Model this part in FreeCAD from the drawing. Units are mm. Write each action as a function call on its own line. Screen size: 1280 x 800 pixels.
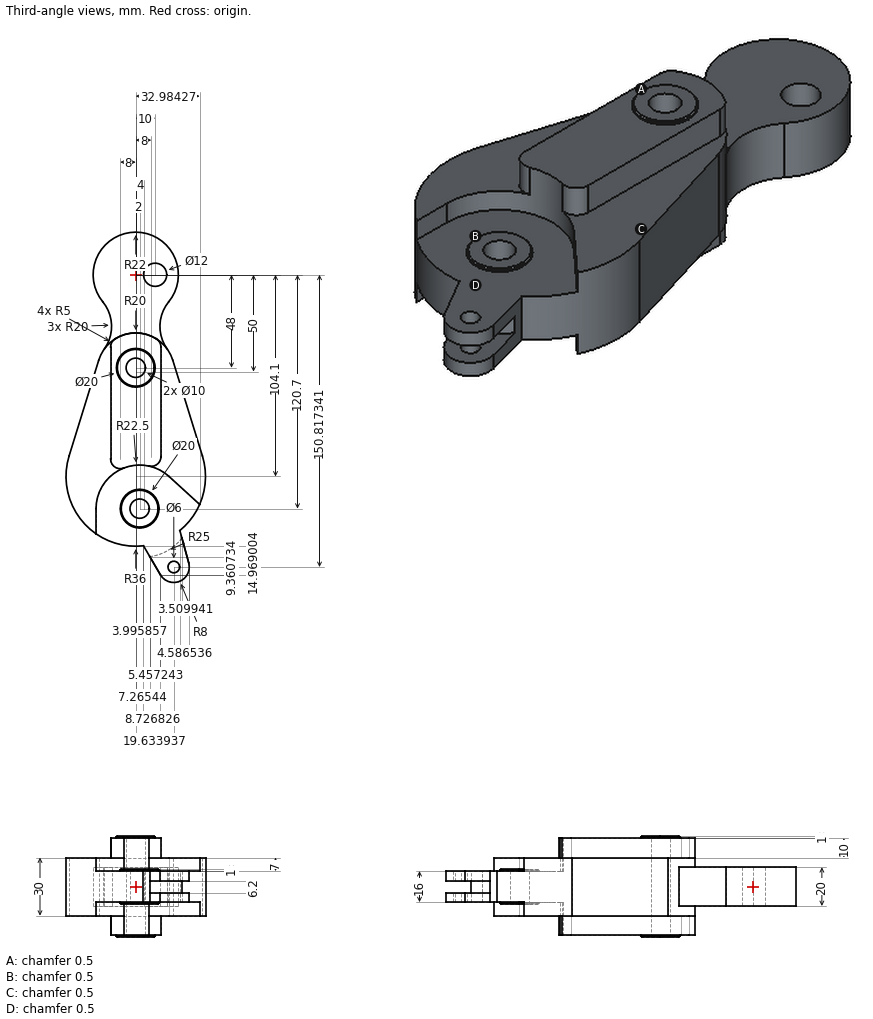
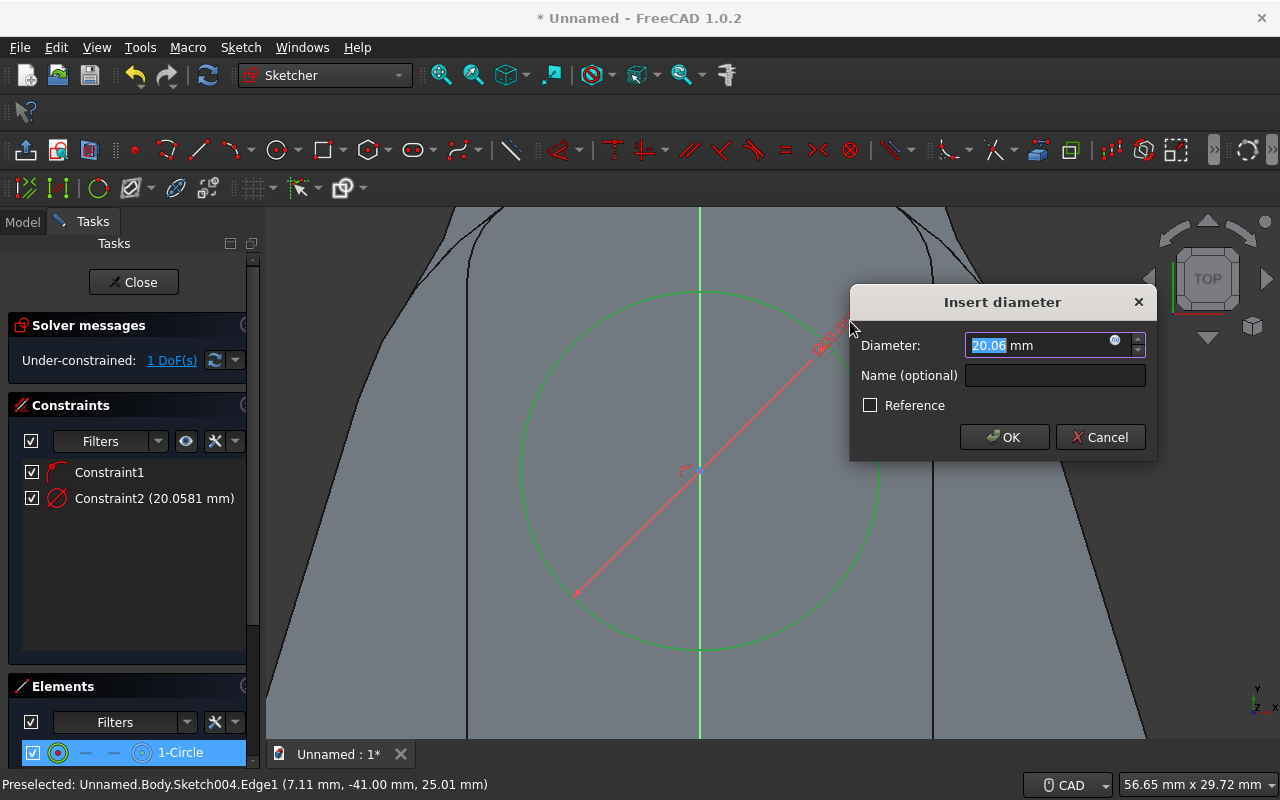
text(20)
key(Return)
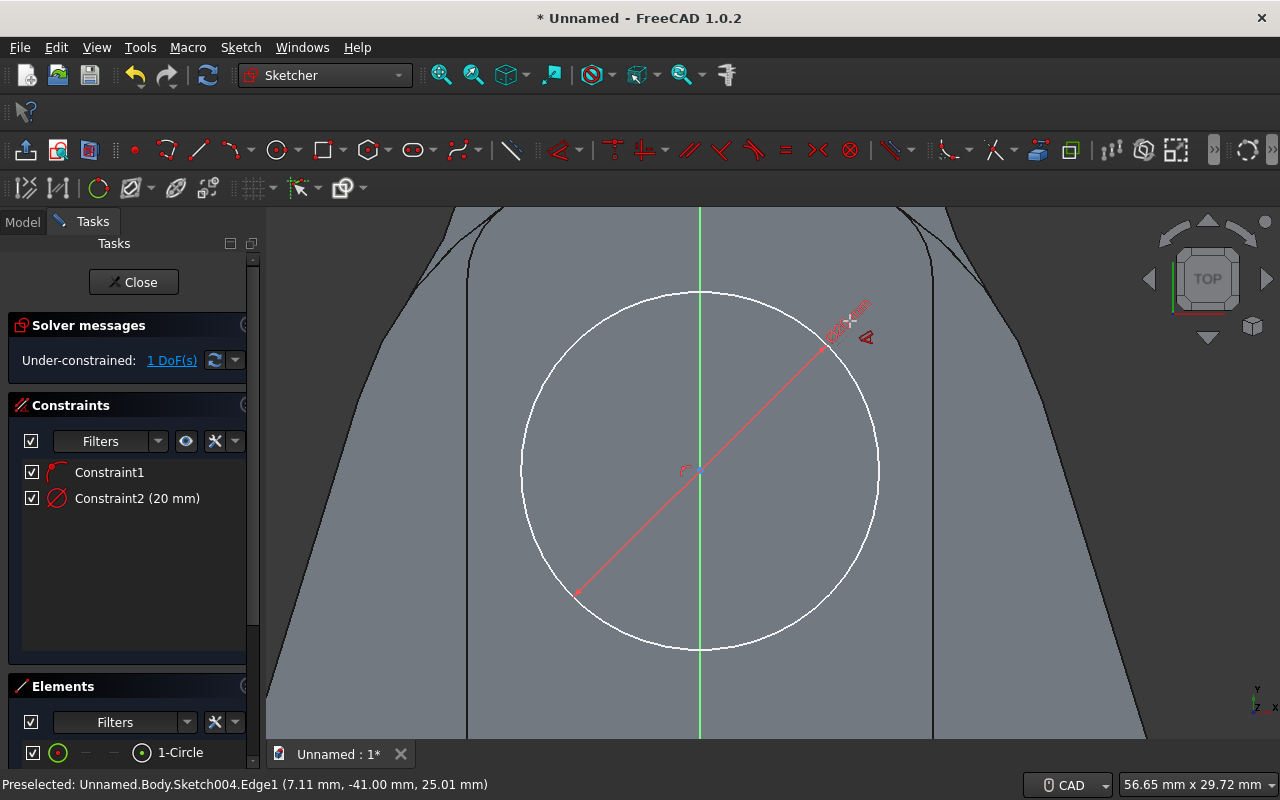
click(700, 471)
click(734, 353)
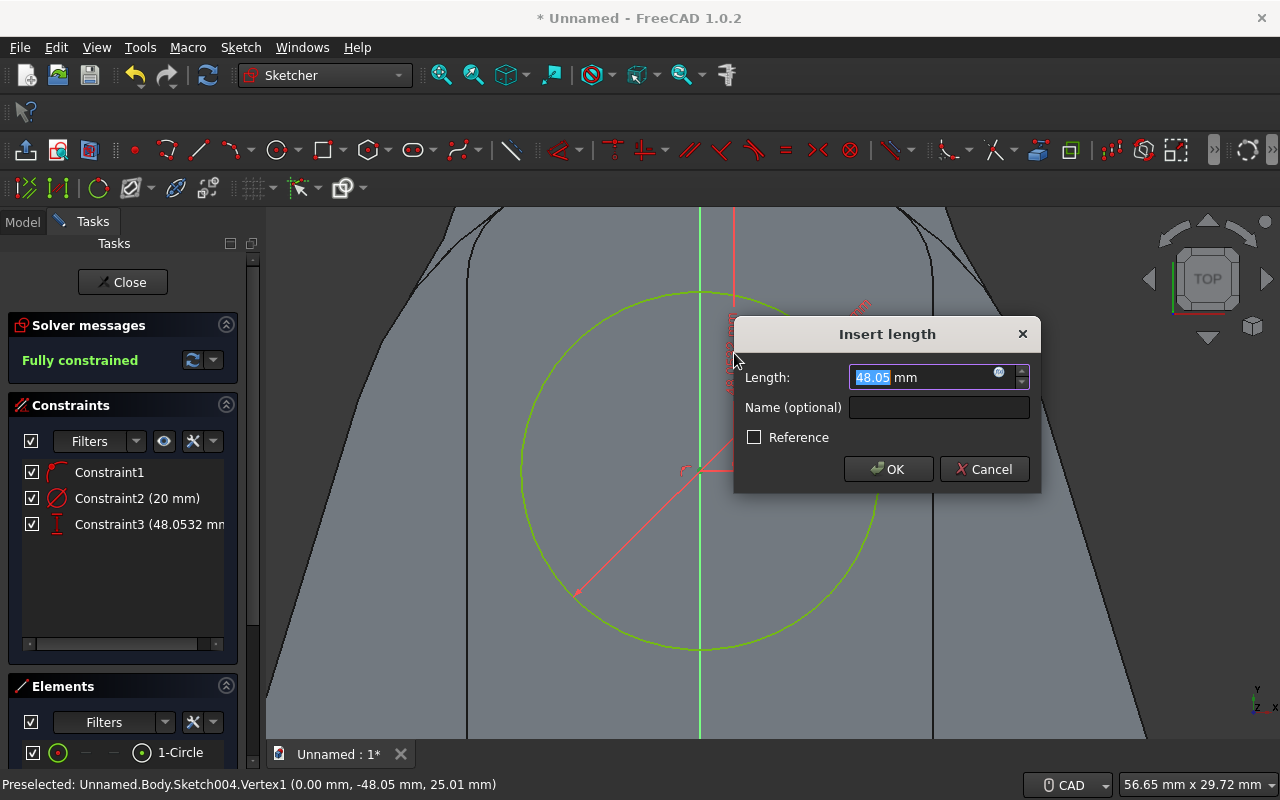
text(48)
key(Return)
key(Escape)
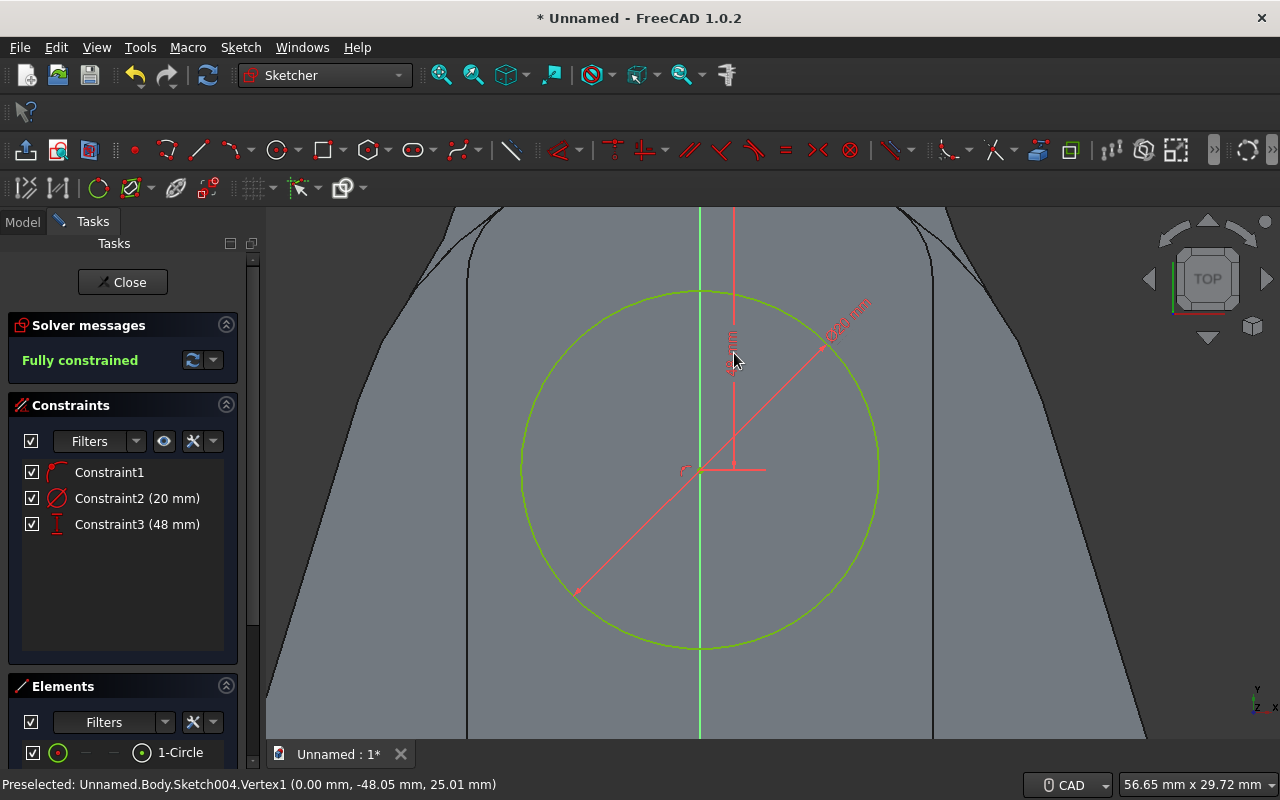
click(123, 282)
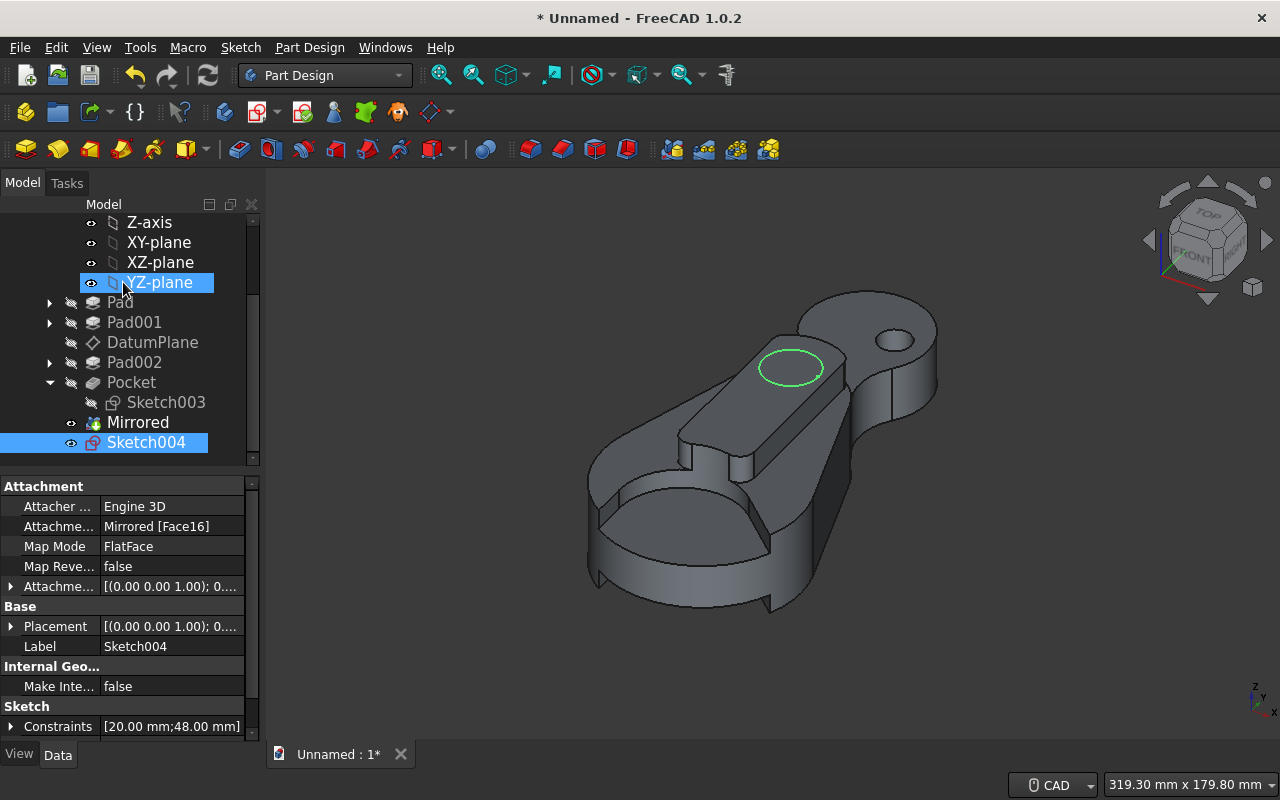
click(26, 150)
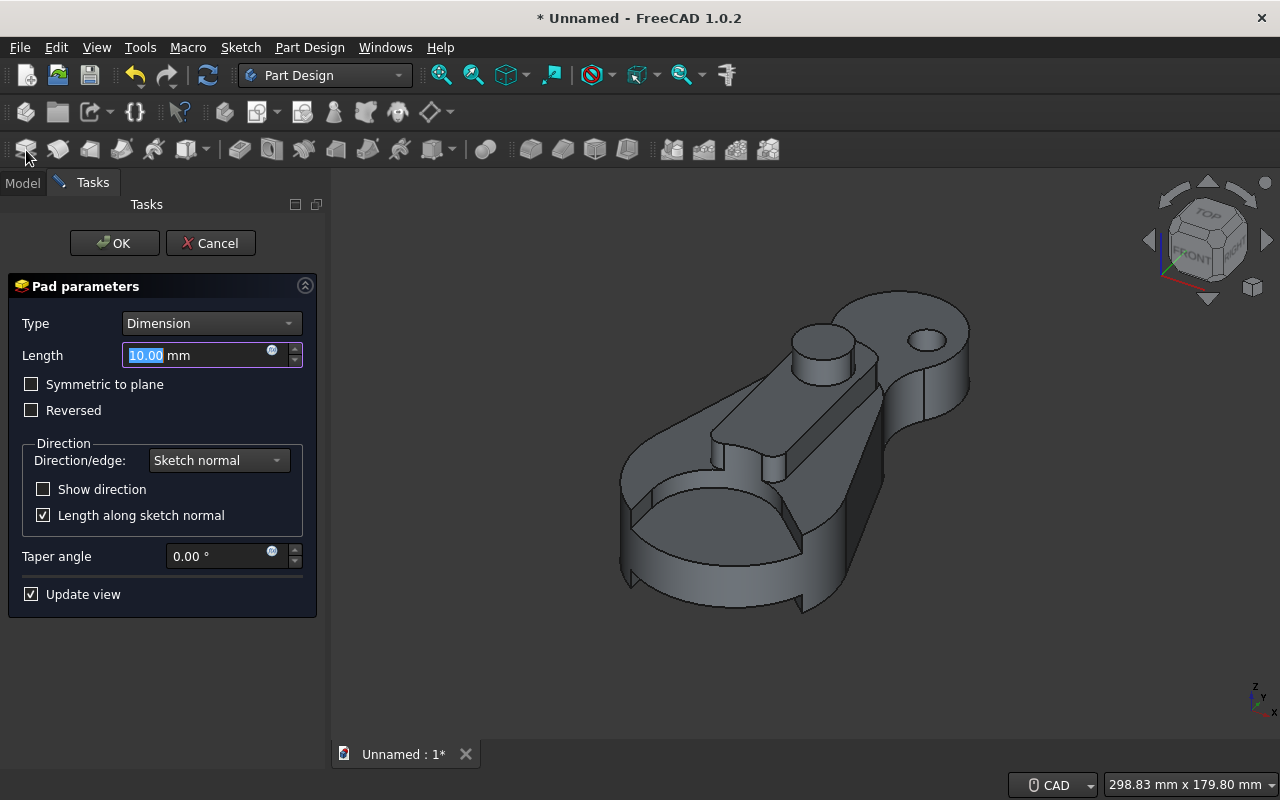
text(1)
key(Tab)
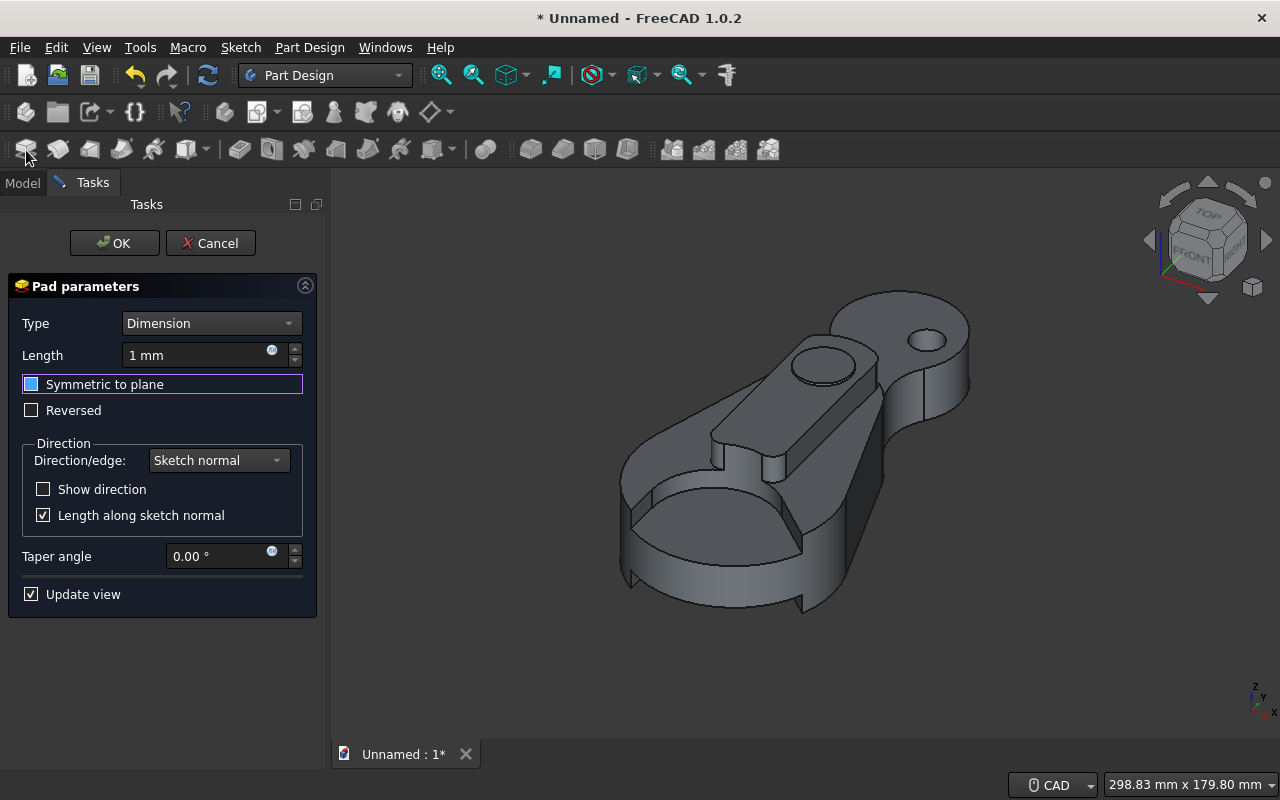
click(115, 243)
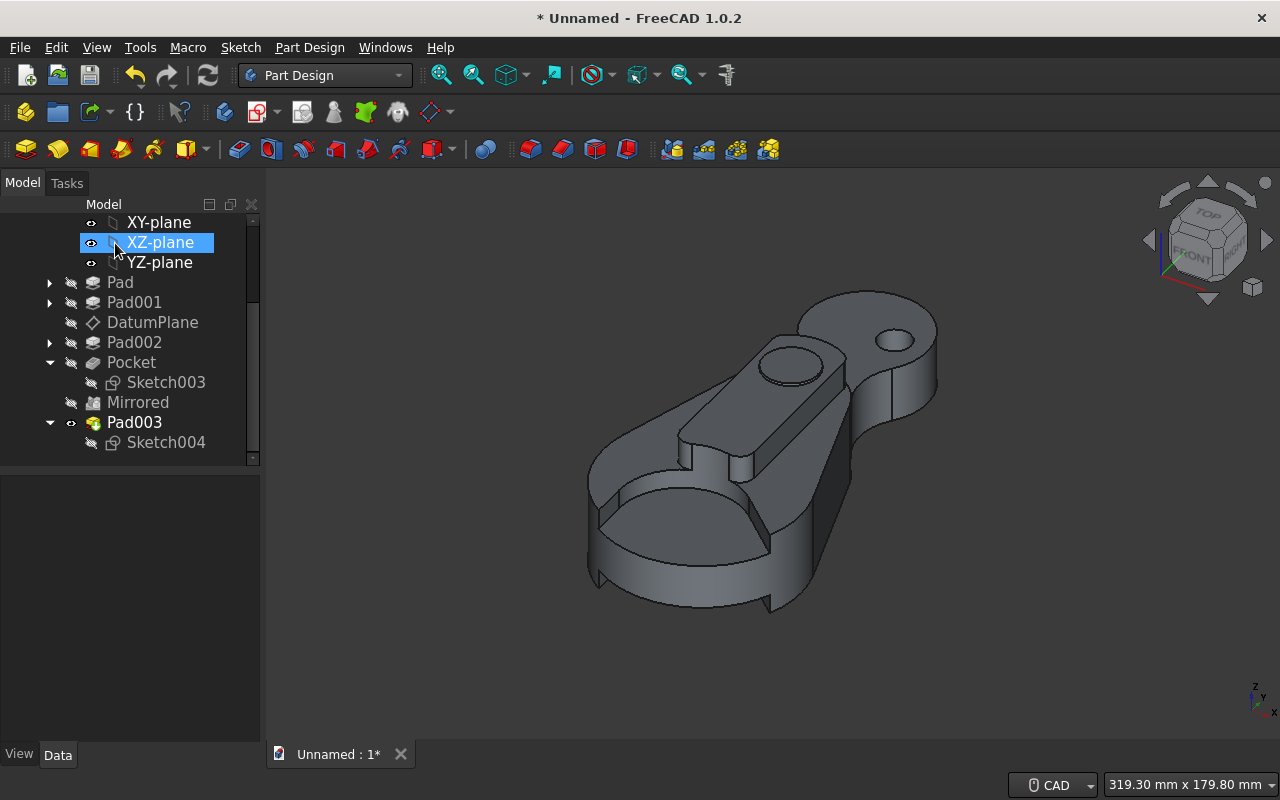
click(759, 366)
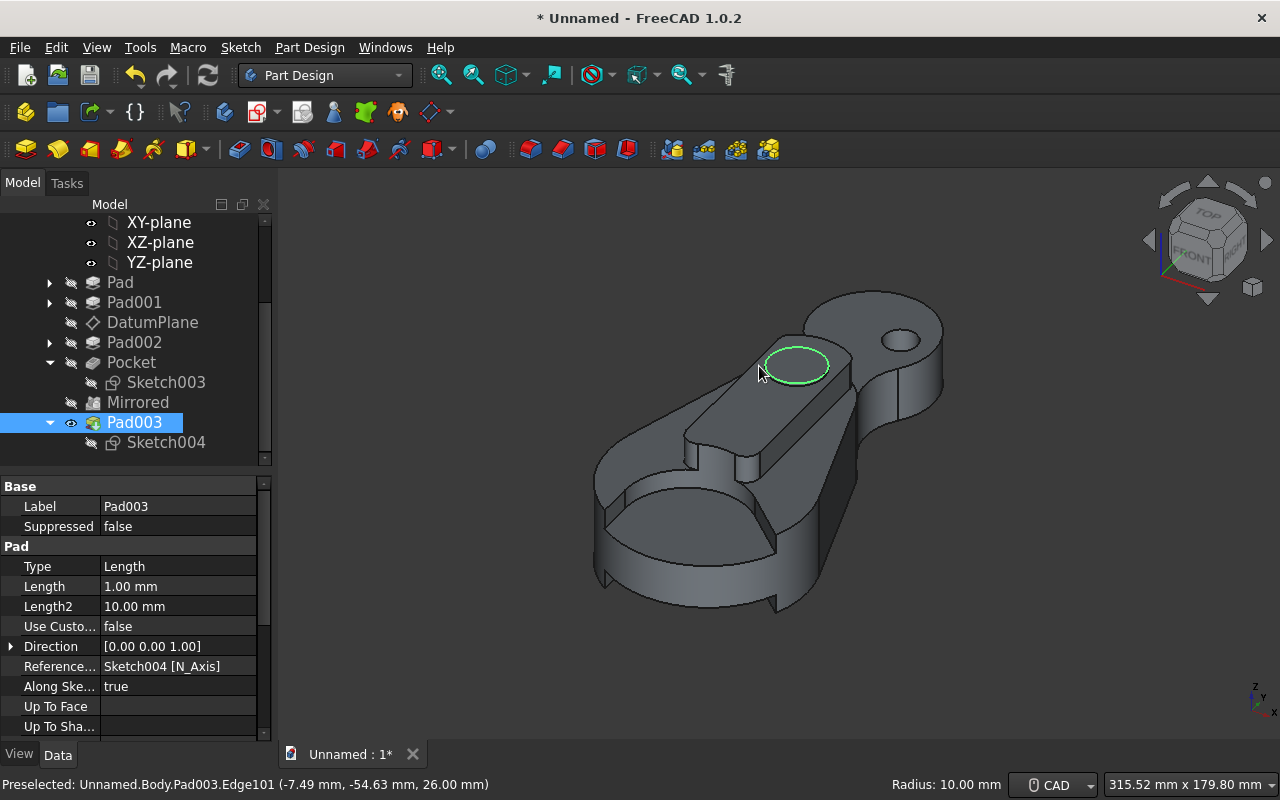
click(564, 150)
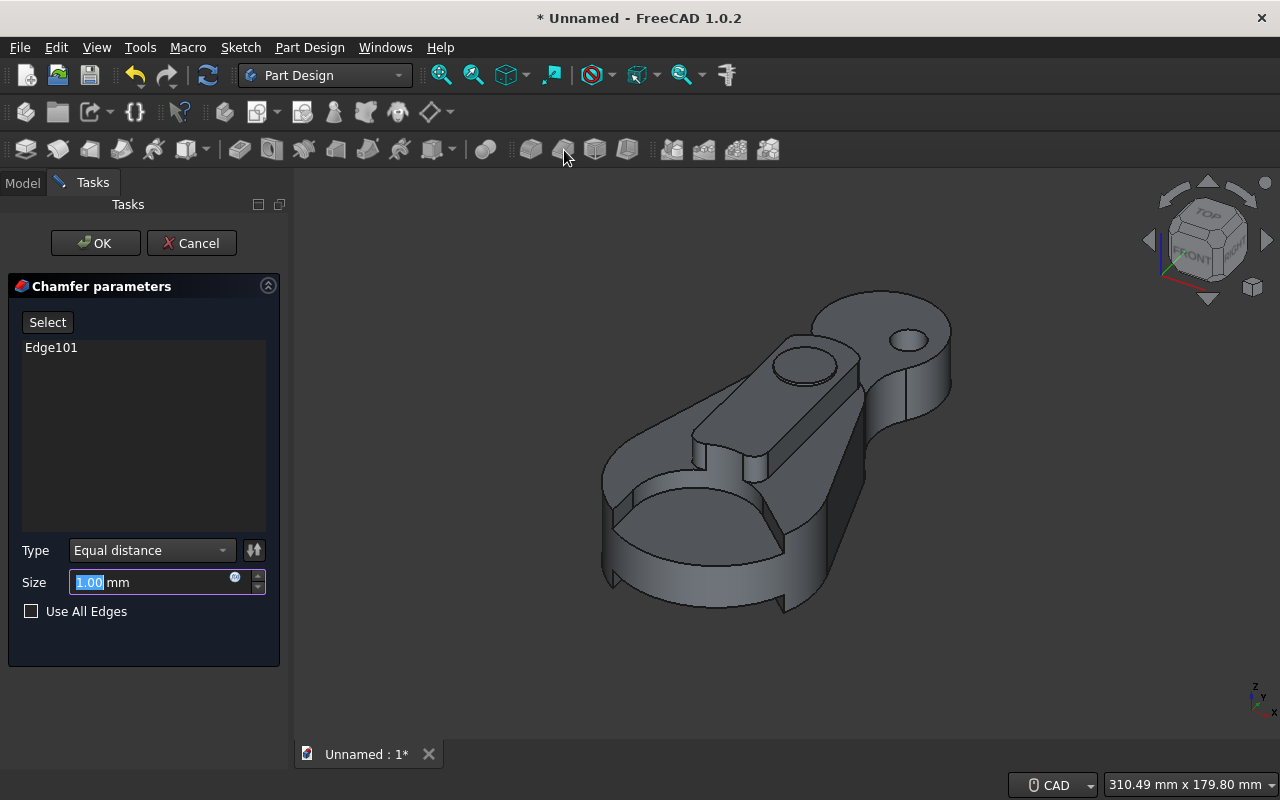
text(0.5)
key(Tab)